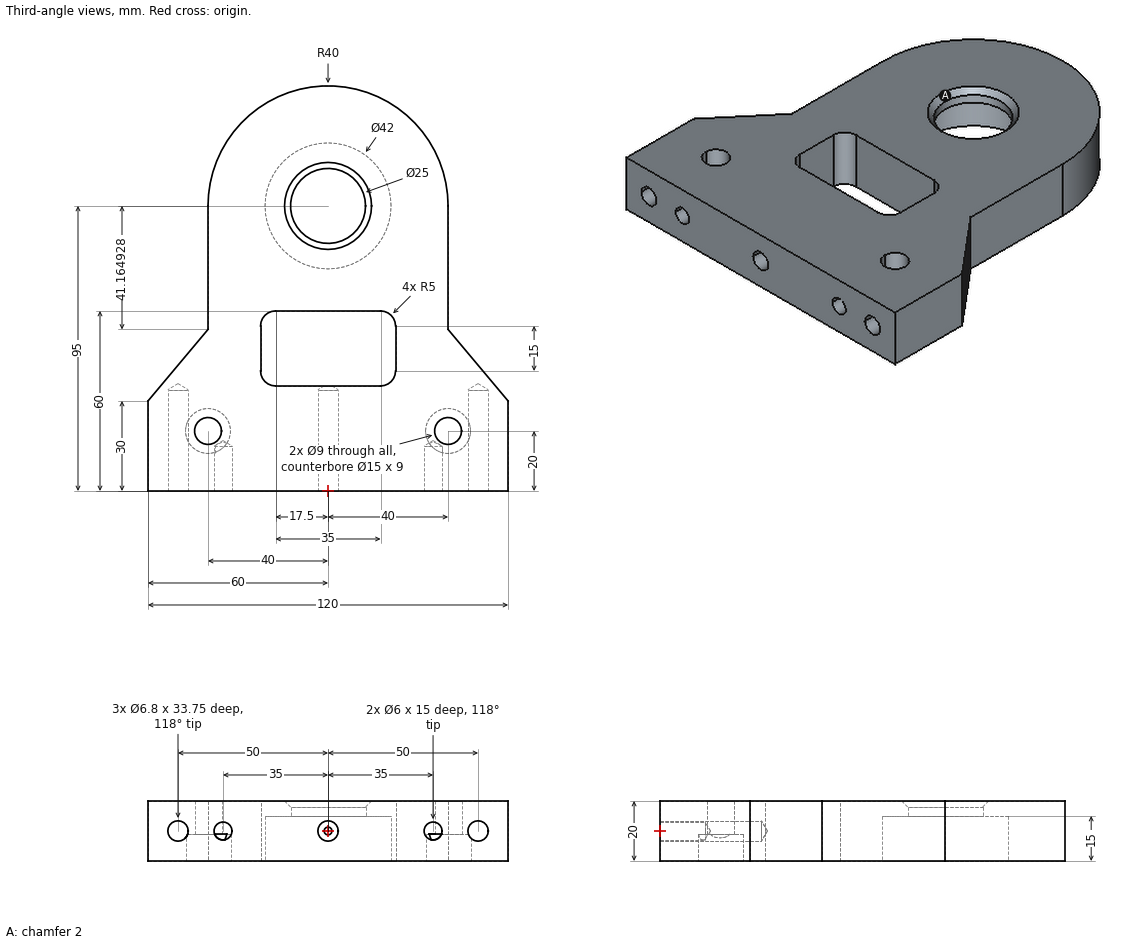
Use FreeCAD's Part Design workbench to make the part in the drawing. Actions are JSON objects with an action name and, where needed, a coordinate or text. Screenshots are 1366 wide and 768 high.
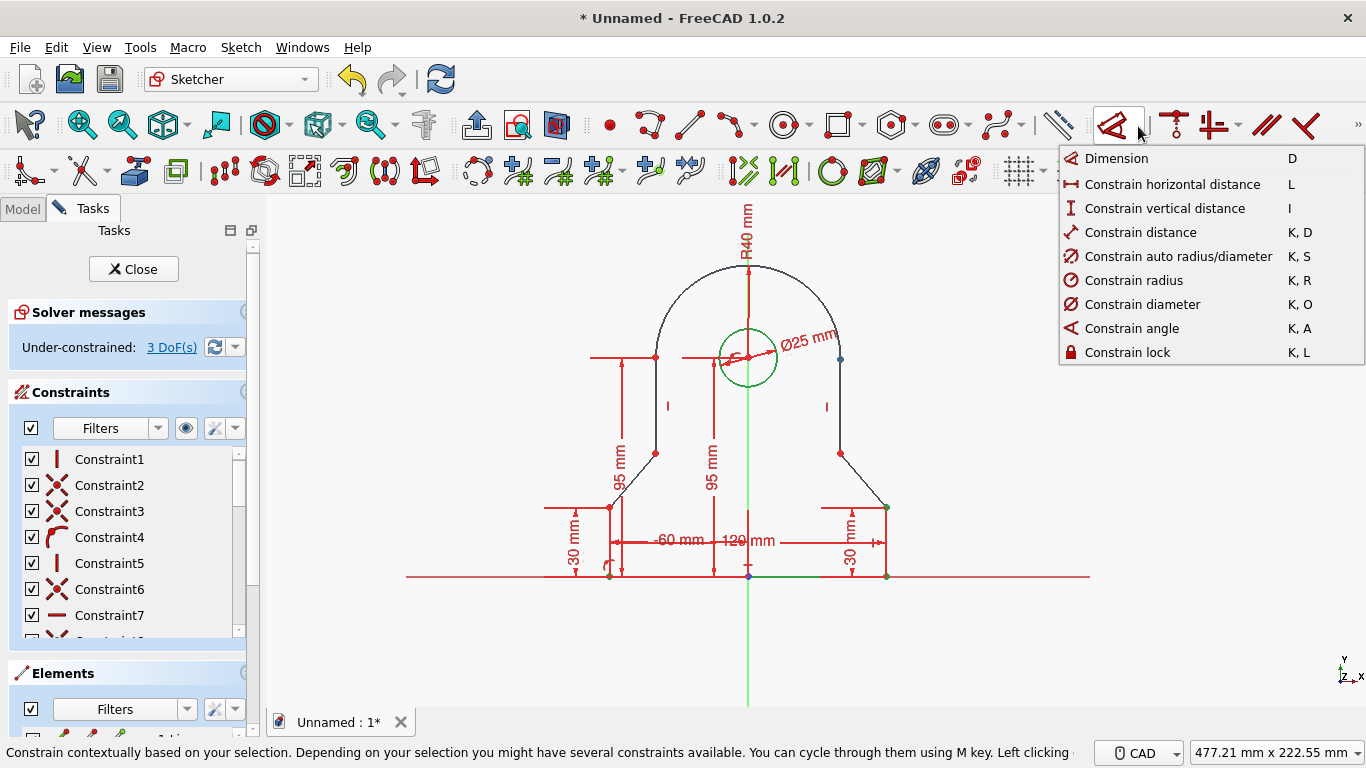
{"action": "left_click", "coordinate": [1212, 208]}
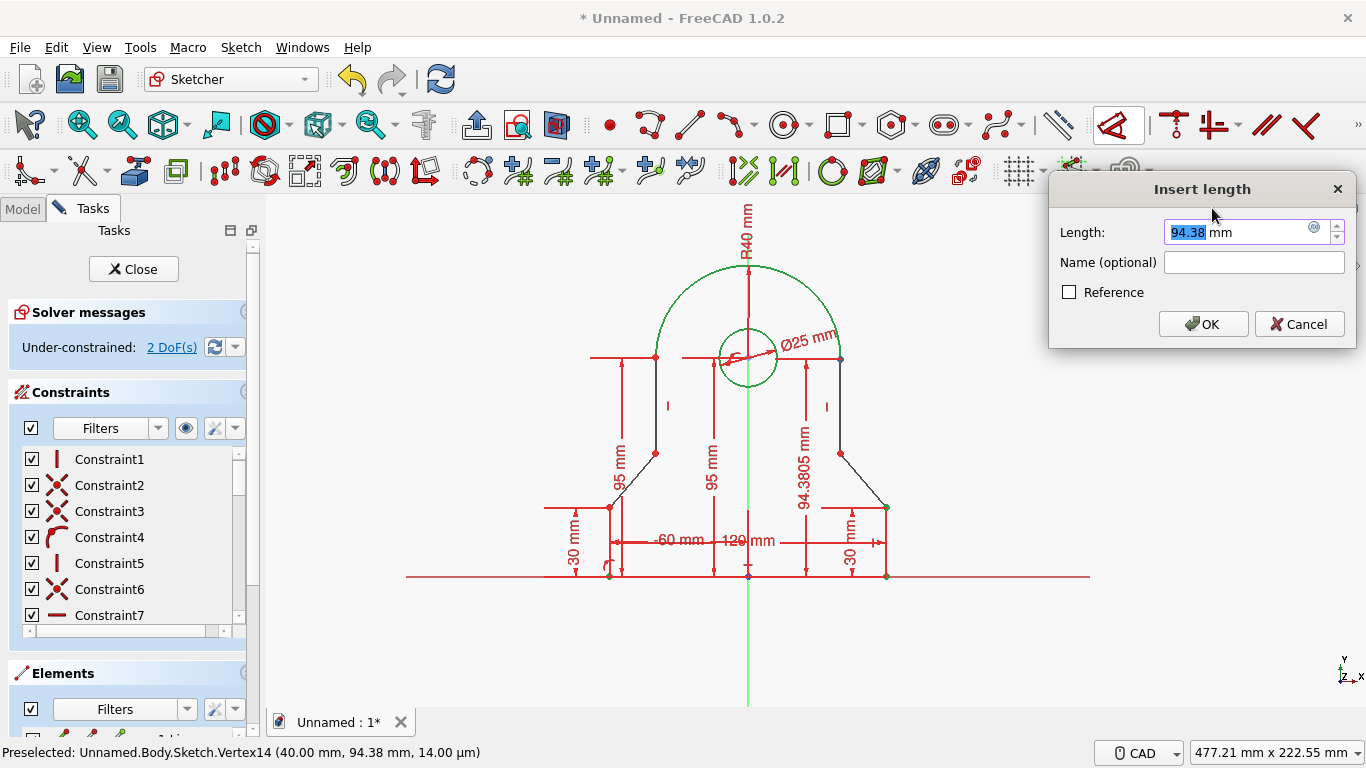
{"action": "type", "text": "95"}
{"action": "key", "text": "Return"}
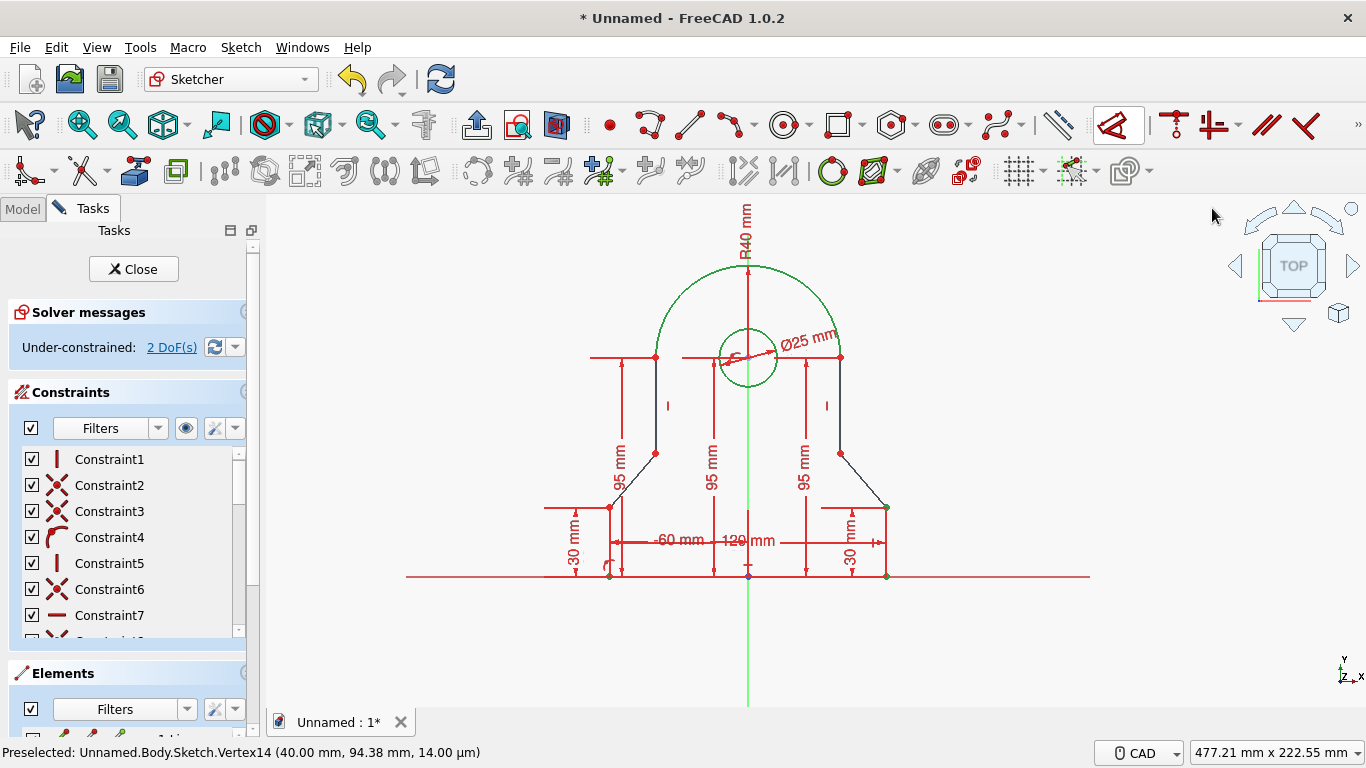
{"action": "left_click", "coordinate": [656, 387]}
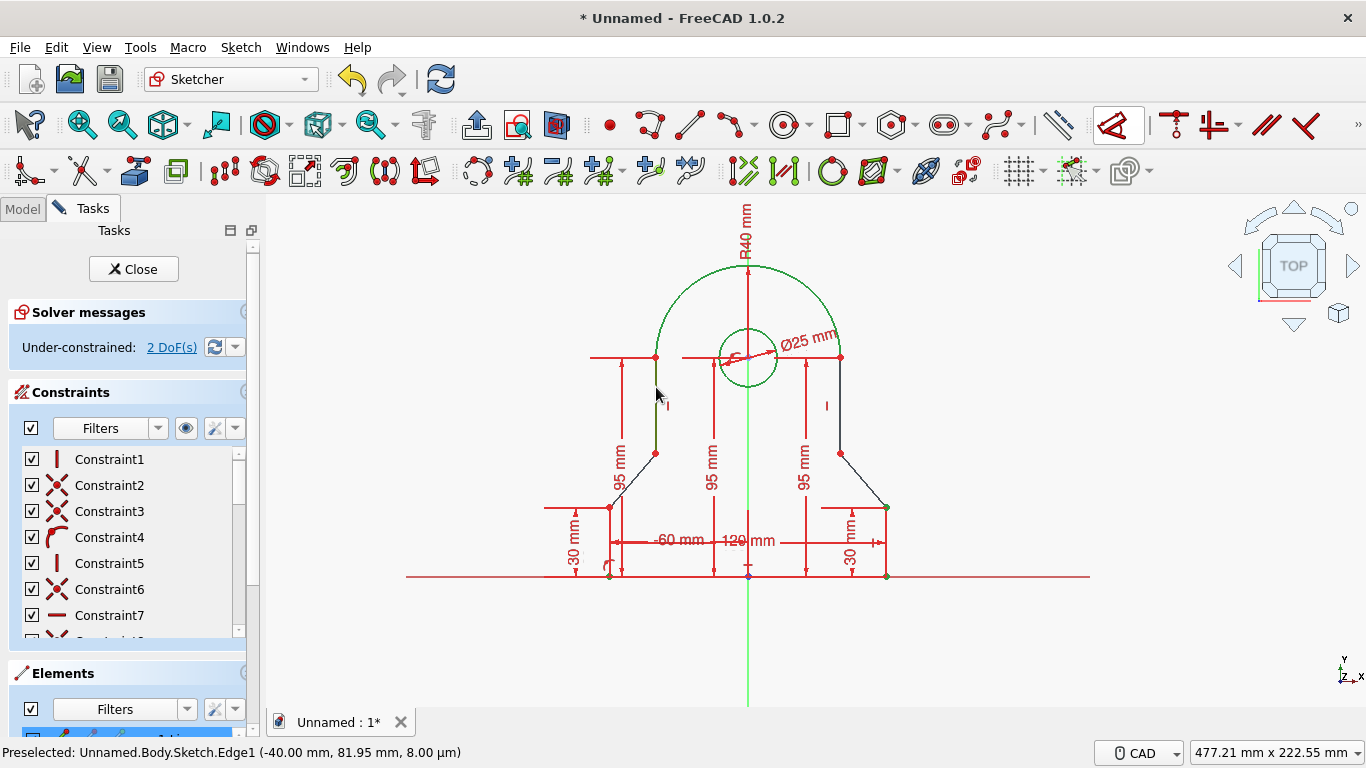
{"action": "left_click", "coordinate": [1138, 126]}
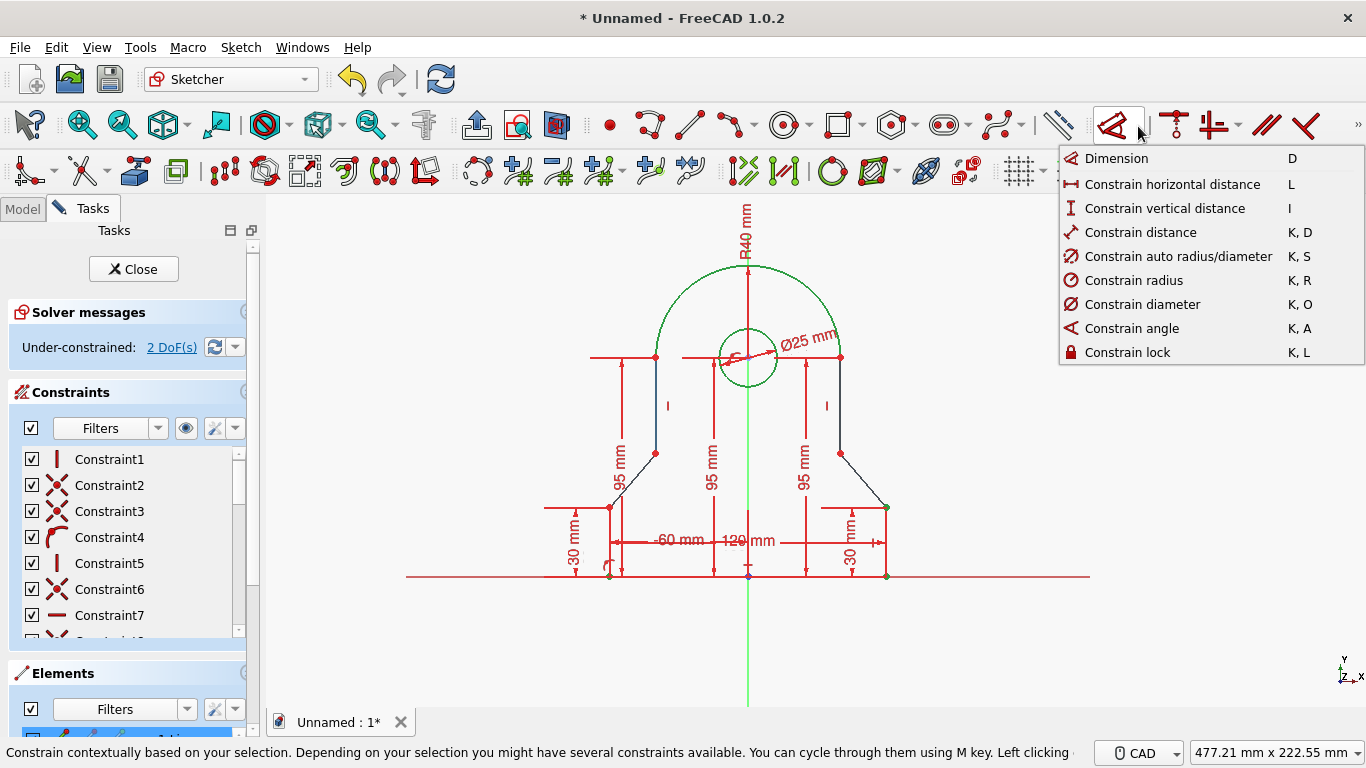
{"action": "left_click", "coordinate": [1212, 208]}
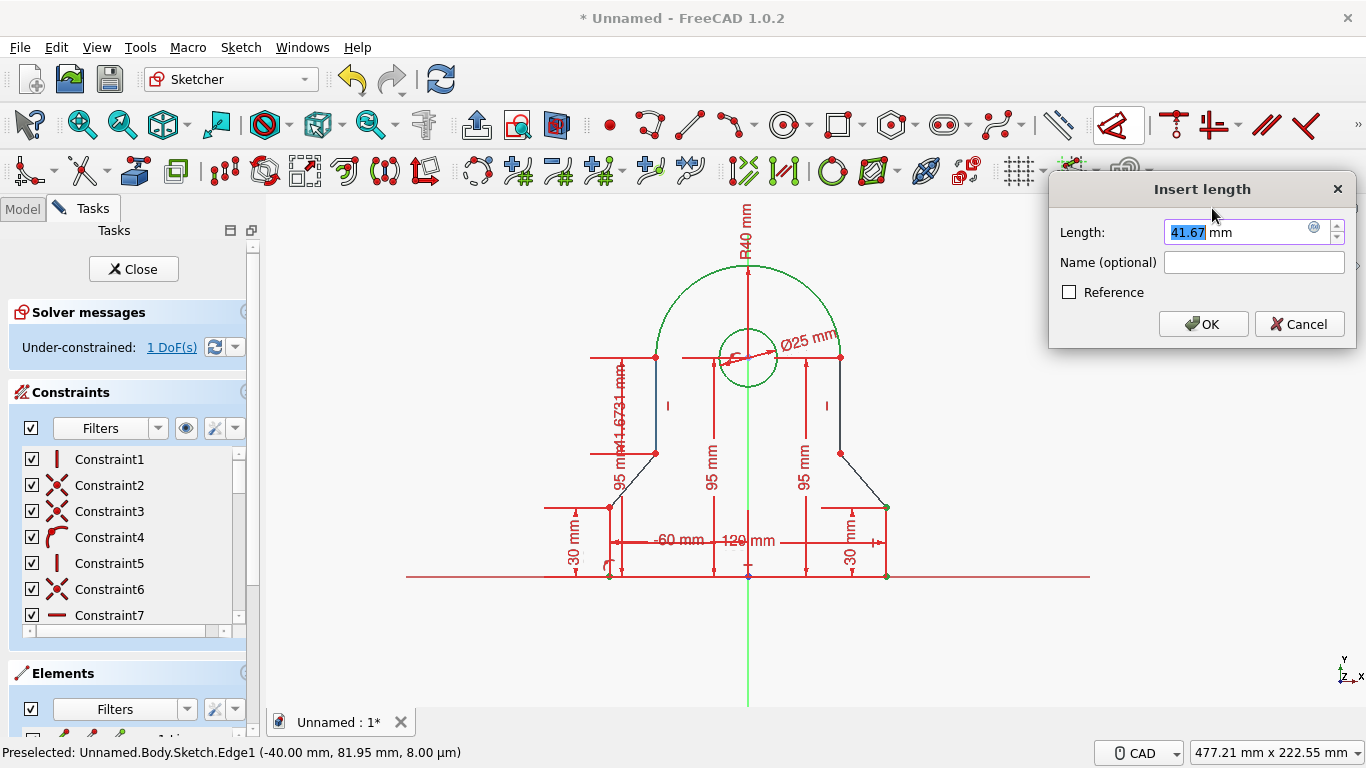
{"action": "type", "text": "41.164928"}
{"action": "key", "text": "Return"}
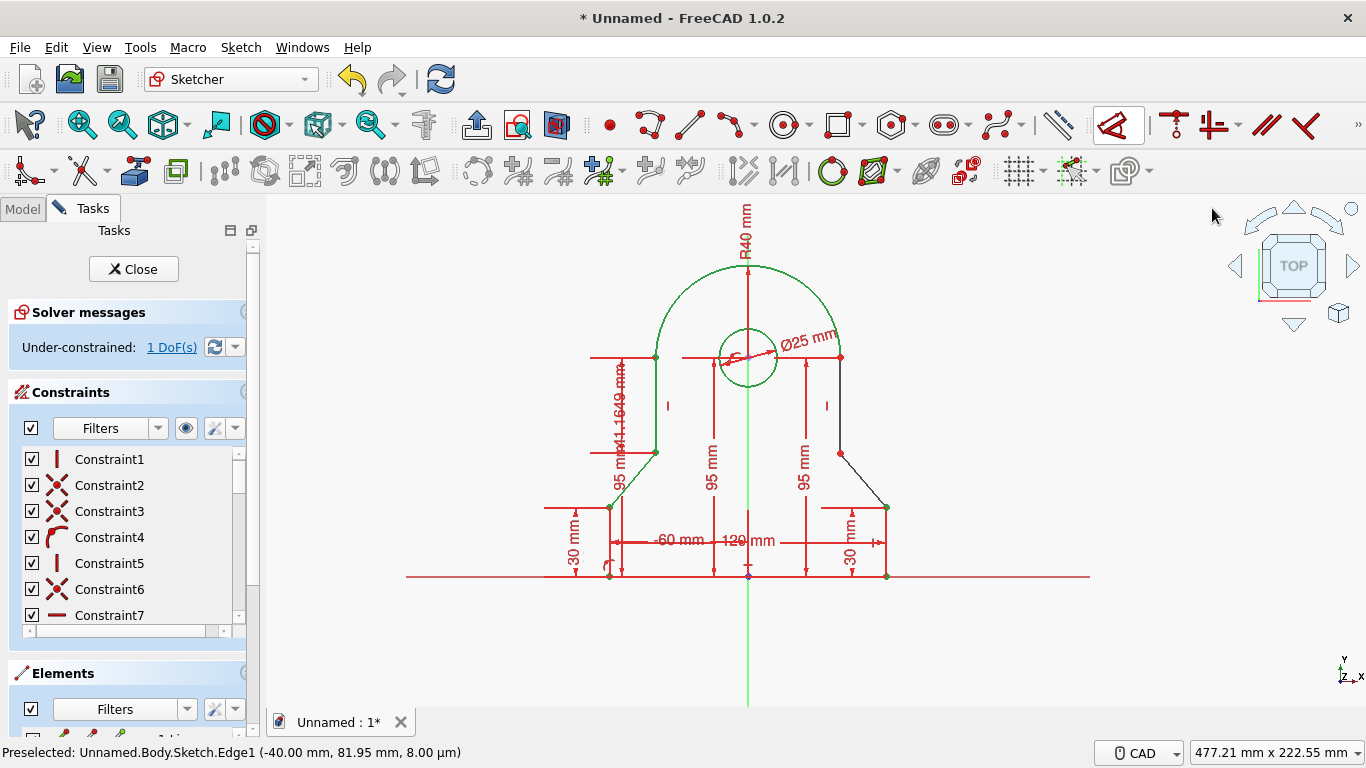
{"action": "left_click", "coordinate": [840, 425]}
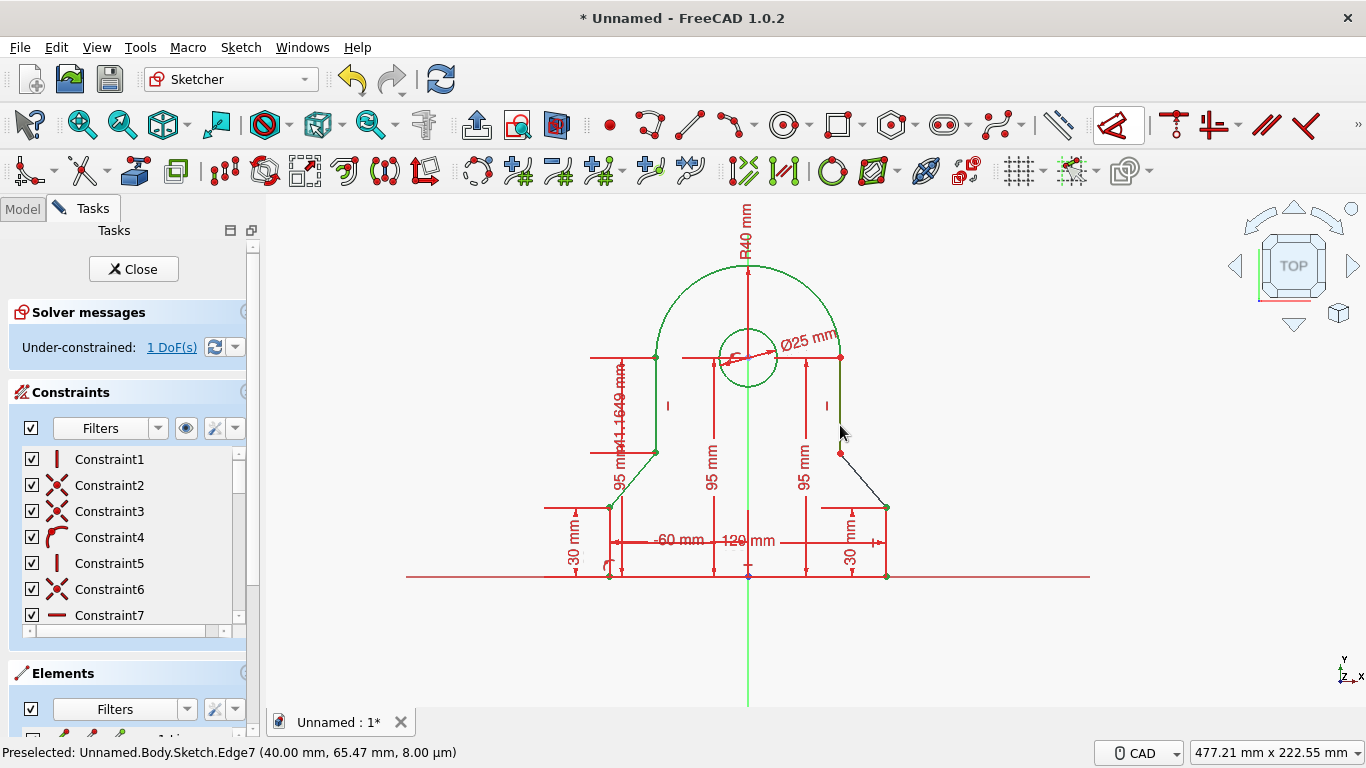
{"action": "left_click", "coordinate": [1138, 126]}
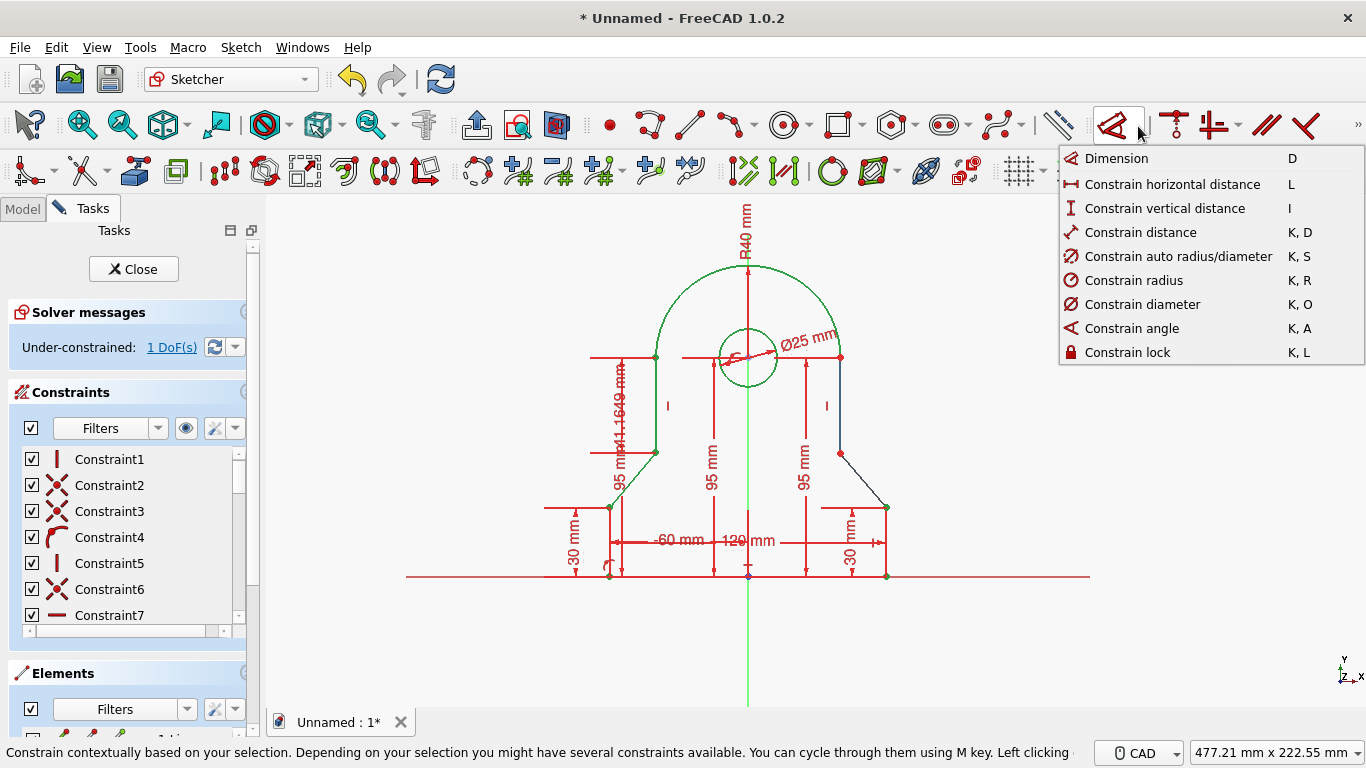
{"action": "left_click", "coordinate": [1212, 208]}